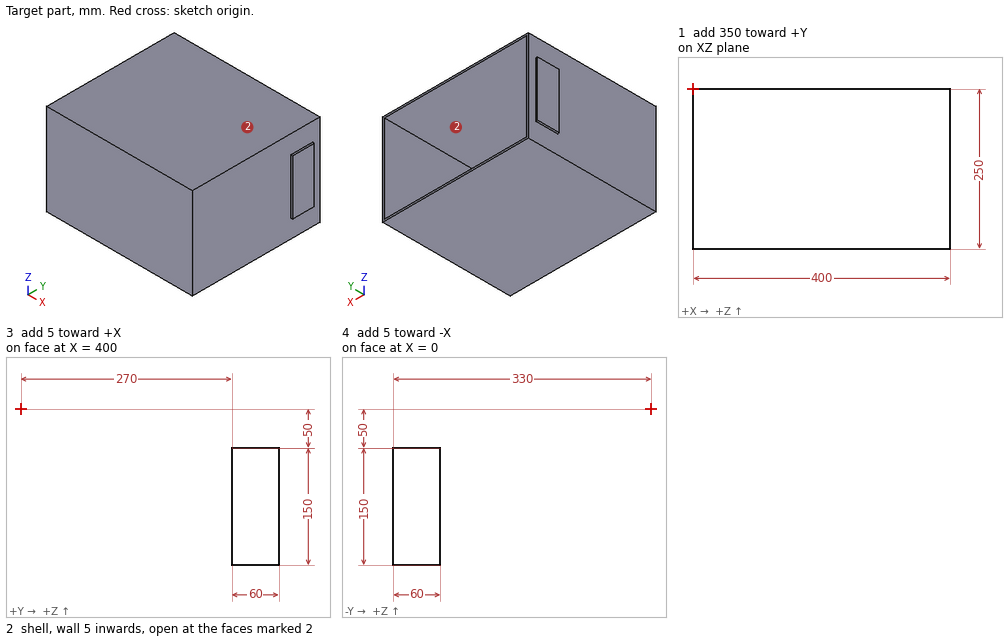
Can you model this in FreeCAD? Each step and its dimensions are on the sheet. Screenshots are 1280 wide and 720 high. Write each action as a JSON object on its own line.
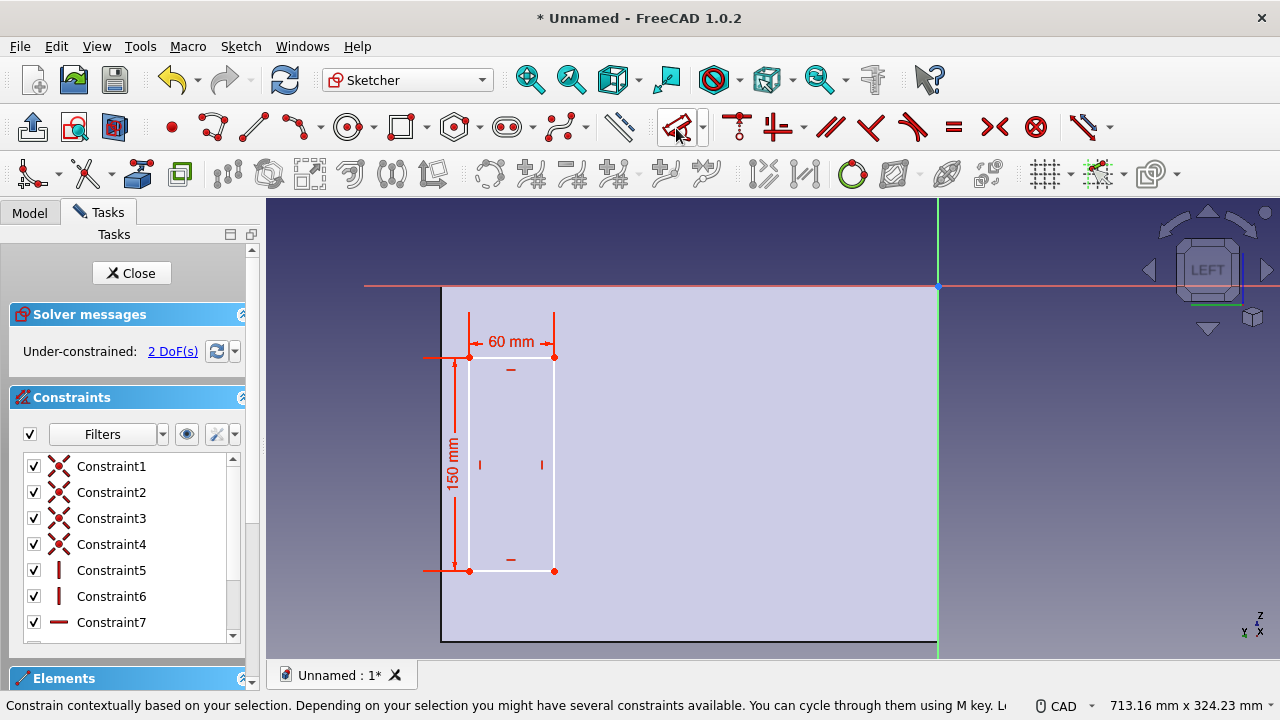
{"action": "left_click", "coordinate": [469, 358]}
{"action": "left_click", "coordinate": [435, 322]}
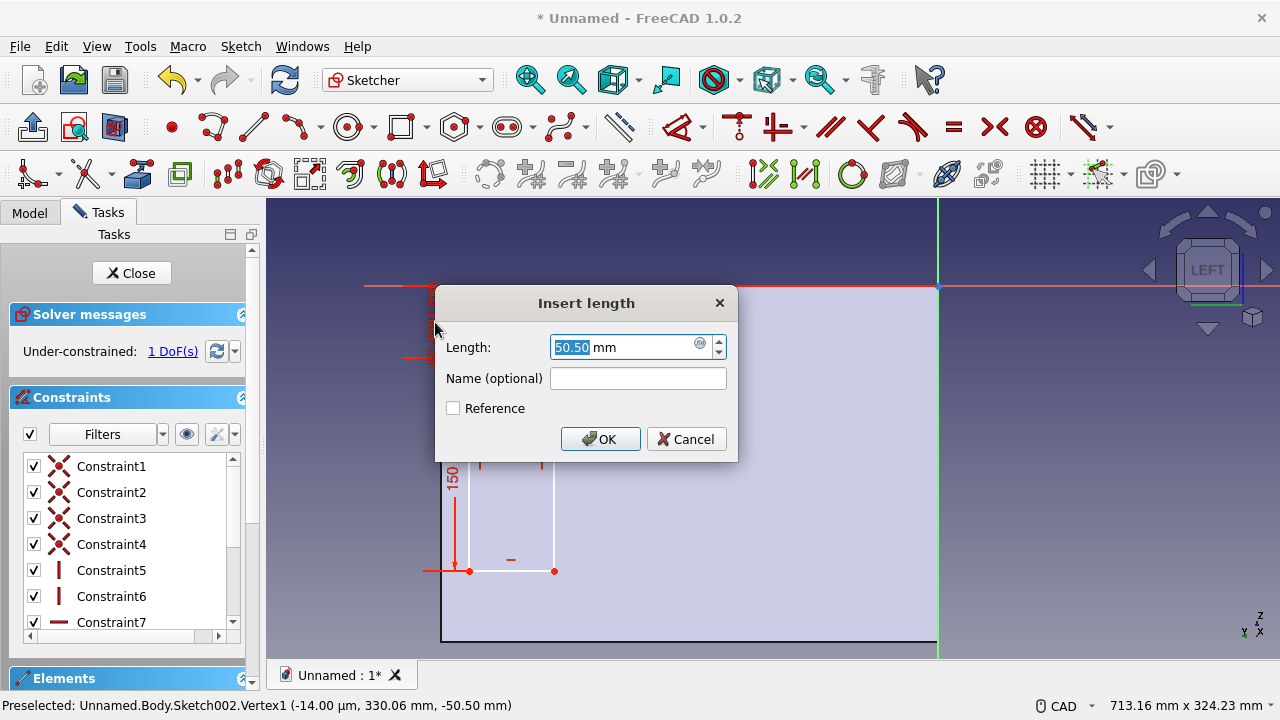
{"action": "type", "text": "50"}
{"action": "key", "text": "Return"}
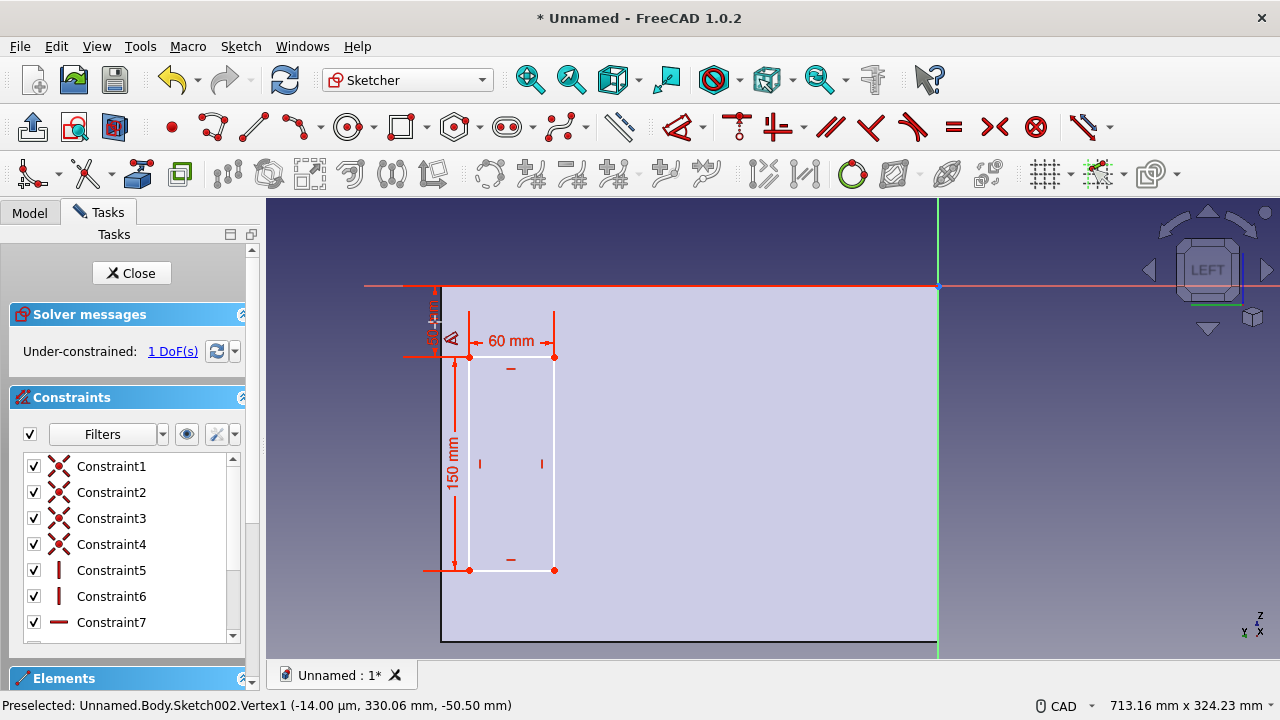
{"action": "left_click", "coordinate": [469, 357]}
{"action": "left_click", "coordinate": [704, 252]}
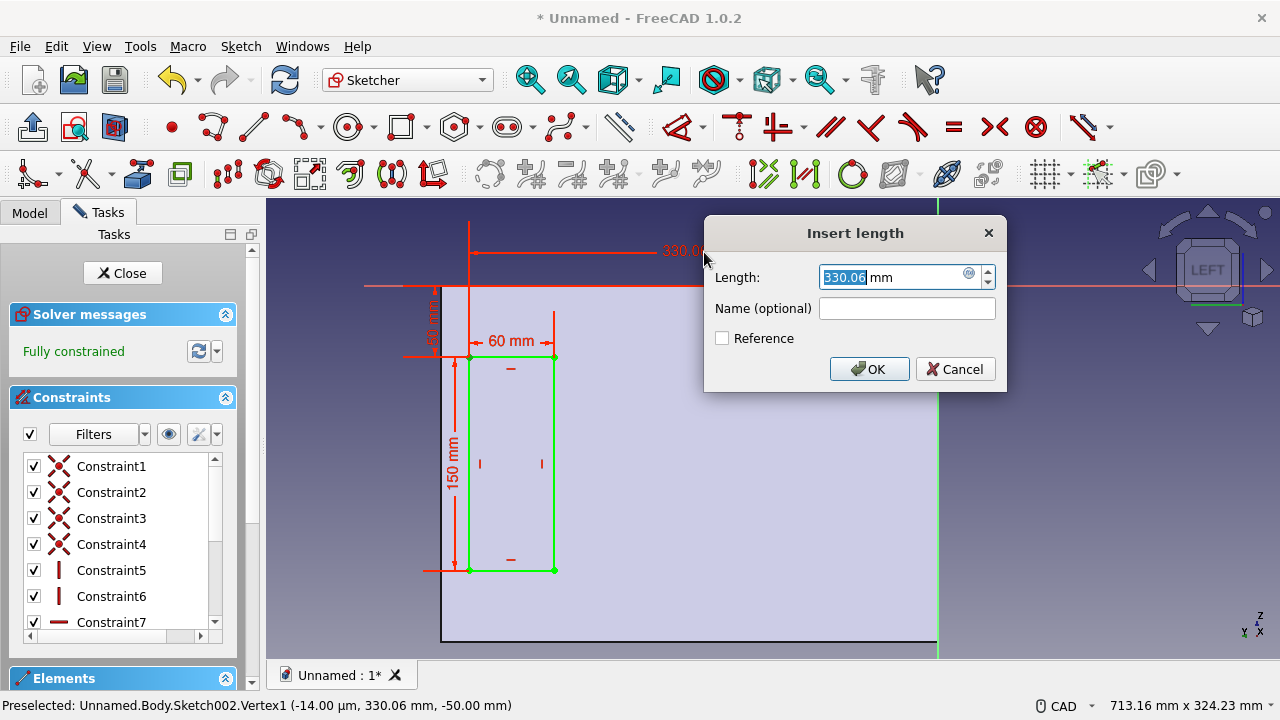
{"action": "type", "text": "330"}
{"action": "key", "text": "Return"}
{"action": "key", "text": "Escape"}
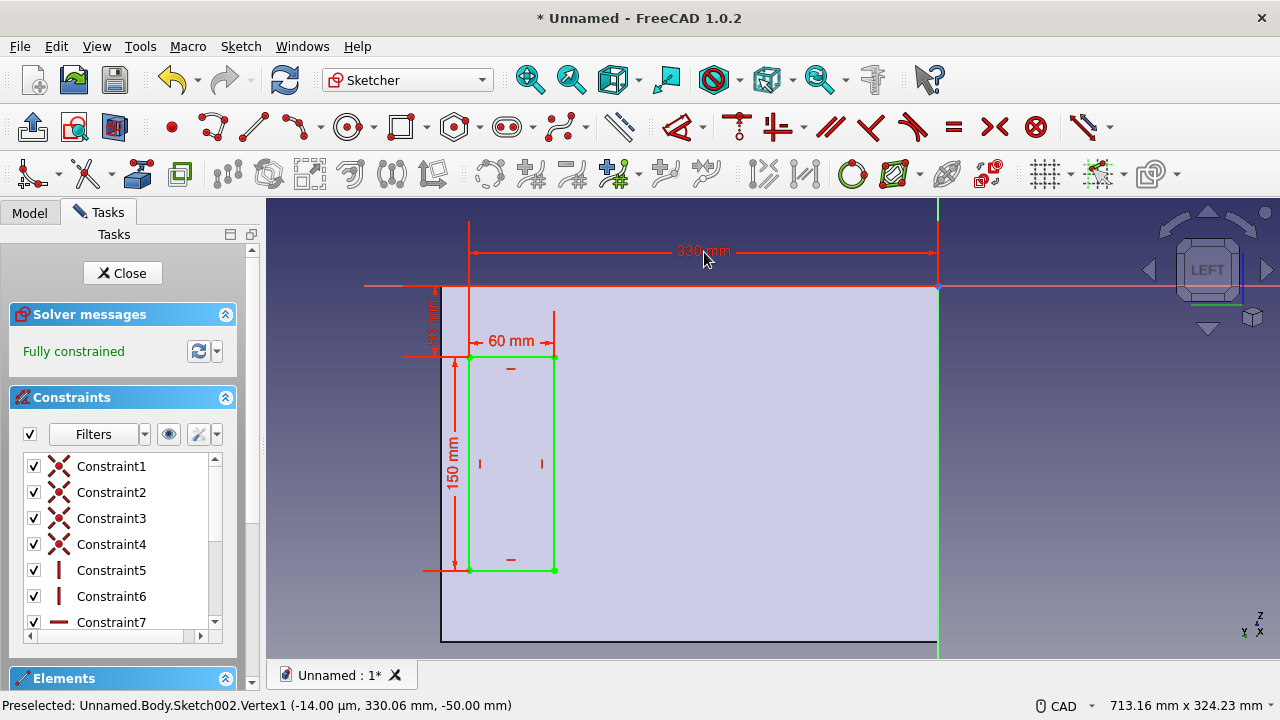
{"action": "left_click", "coordinate": [123, 273]}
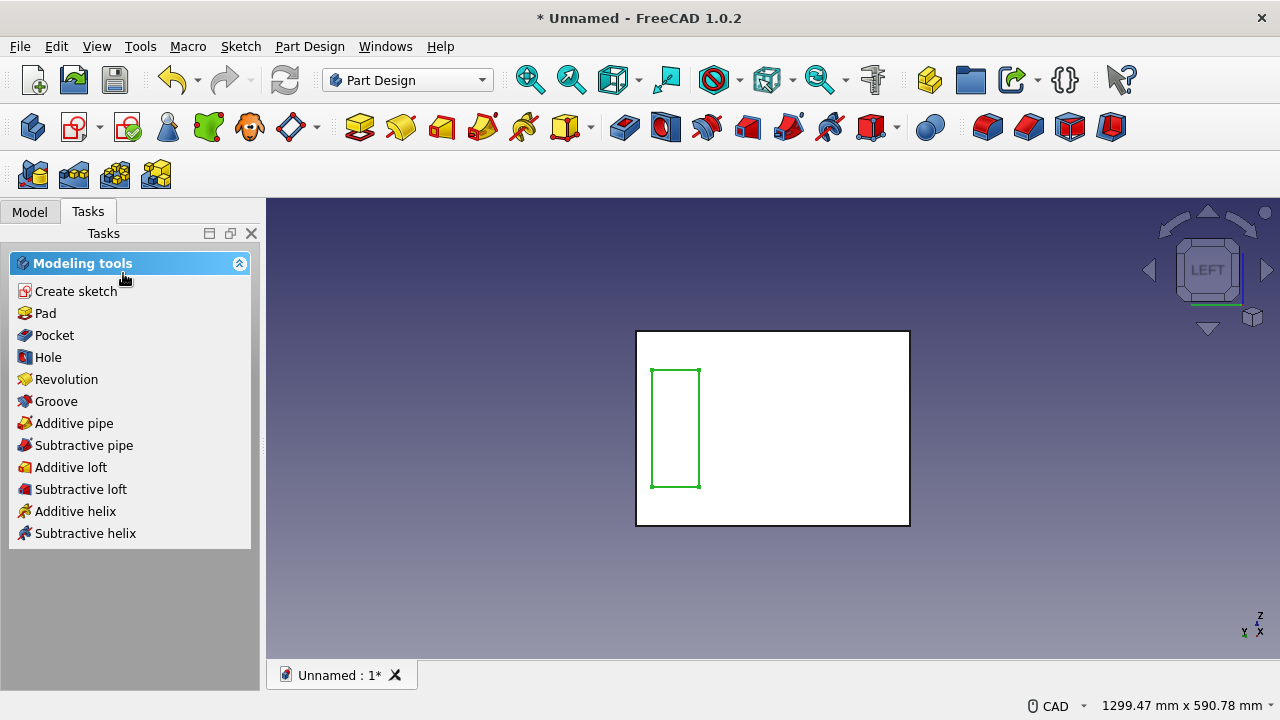
{"action": "left_click", "coordinate": [360, 128]}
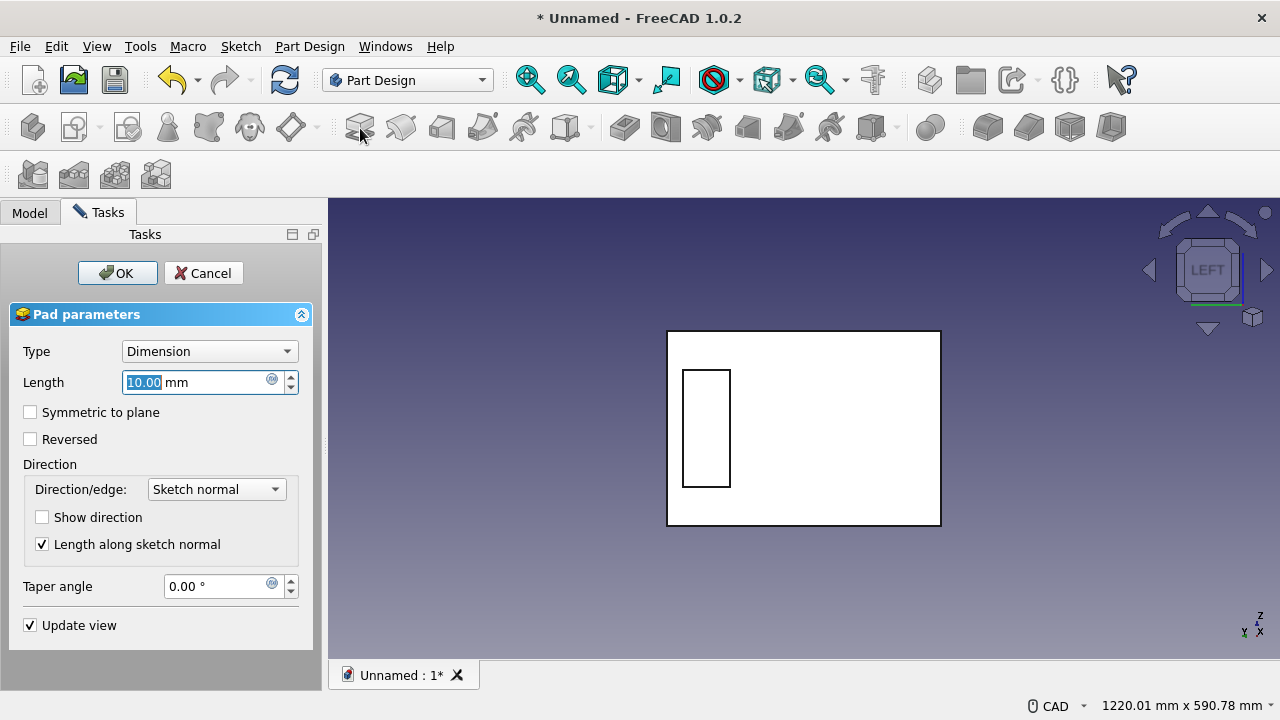
{"action": "type", "text": "5"}
{"action": "key", "text": "Tab"}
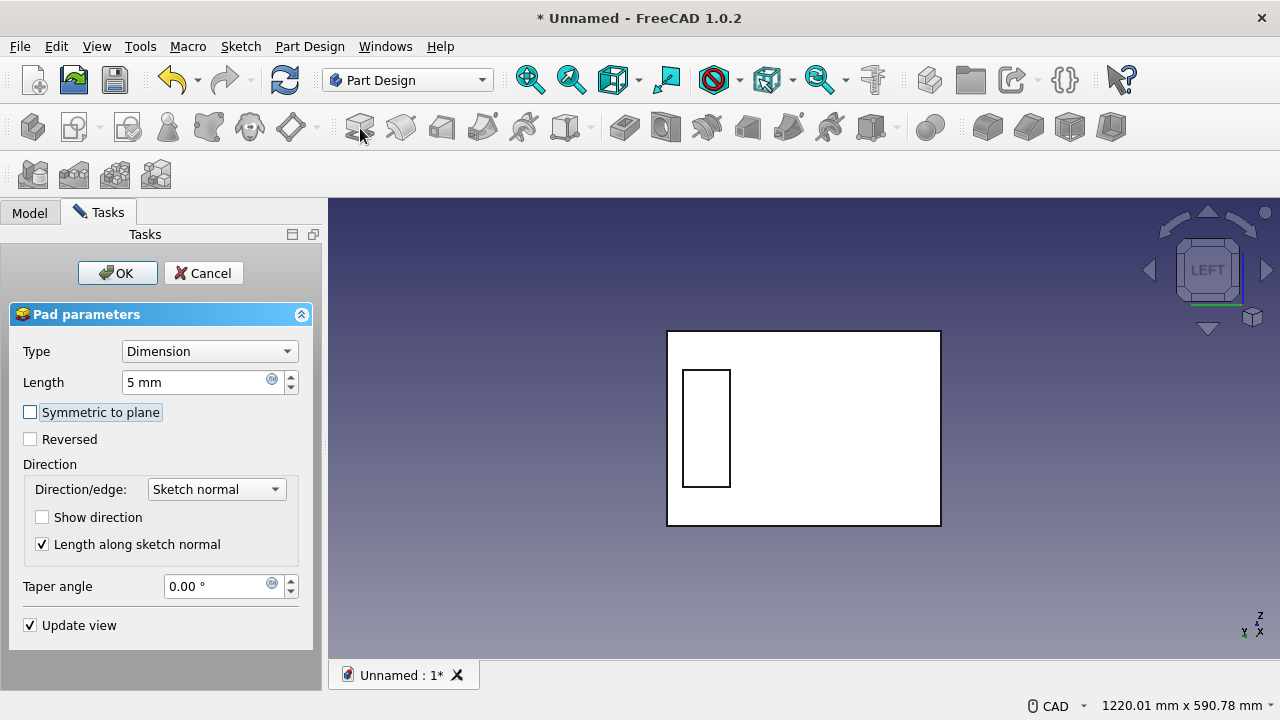
{"action": "left_click", "coordinate": [118, 273]}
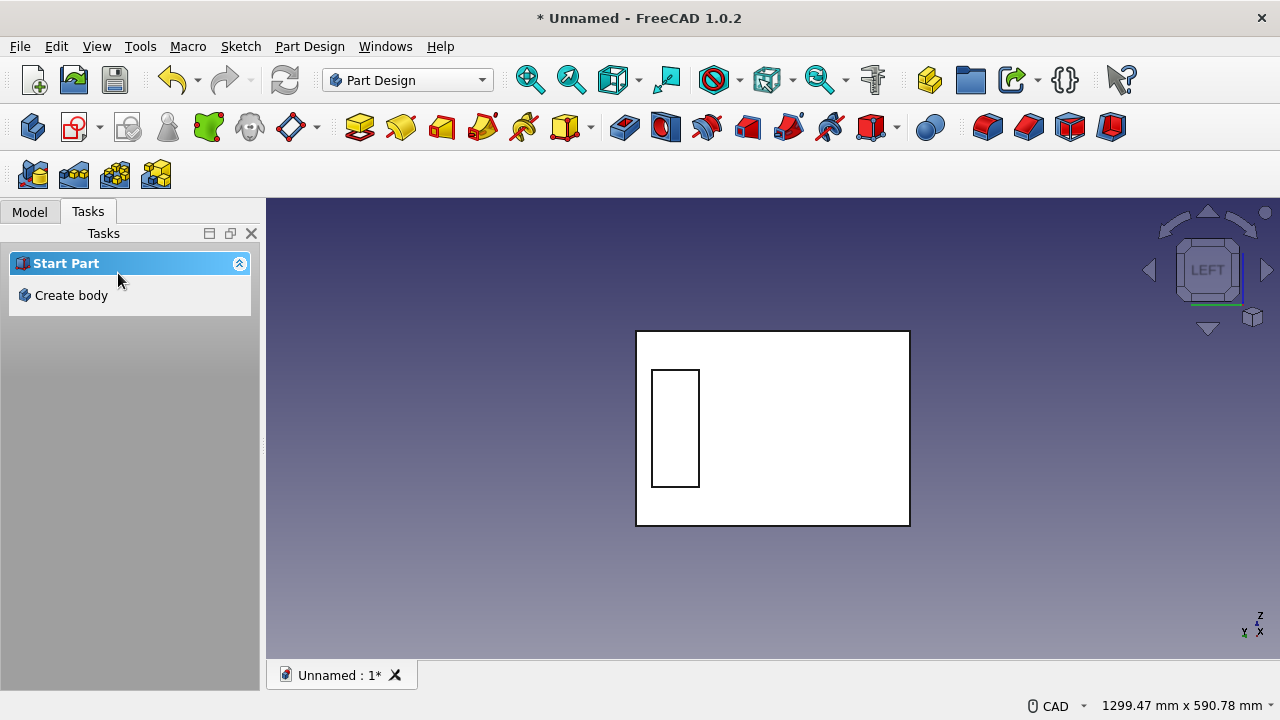
{"action": "key", "text": "0"}